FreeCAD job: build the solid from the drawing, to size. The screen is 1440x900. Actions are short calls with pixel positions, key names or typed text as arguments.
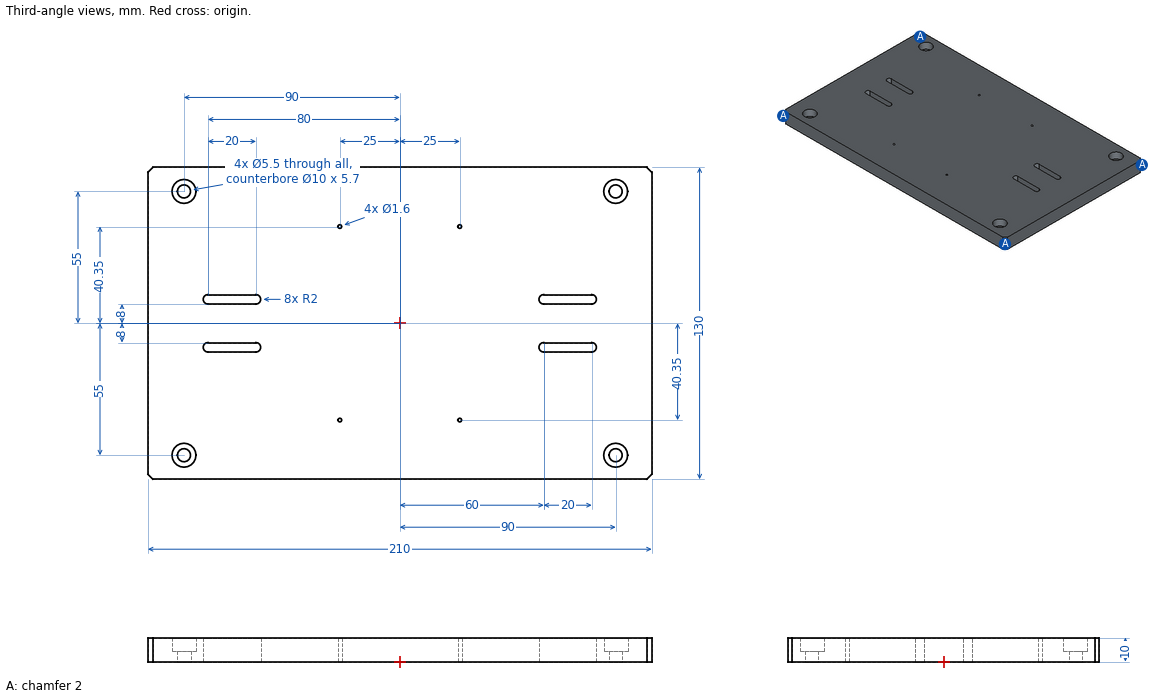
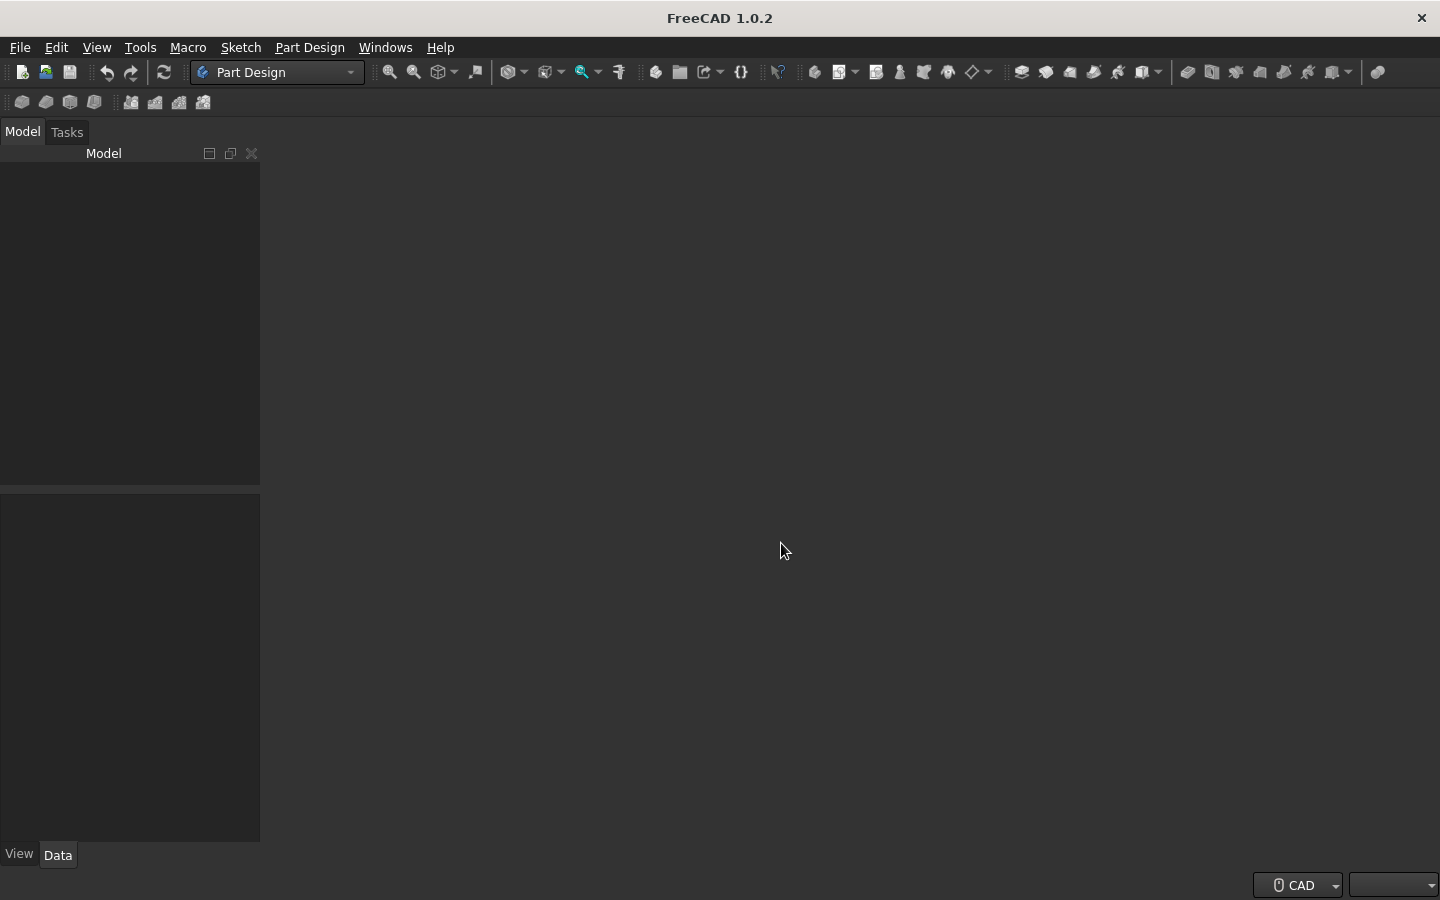
click(22, 72)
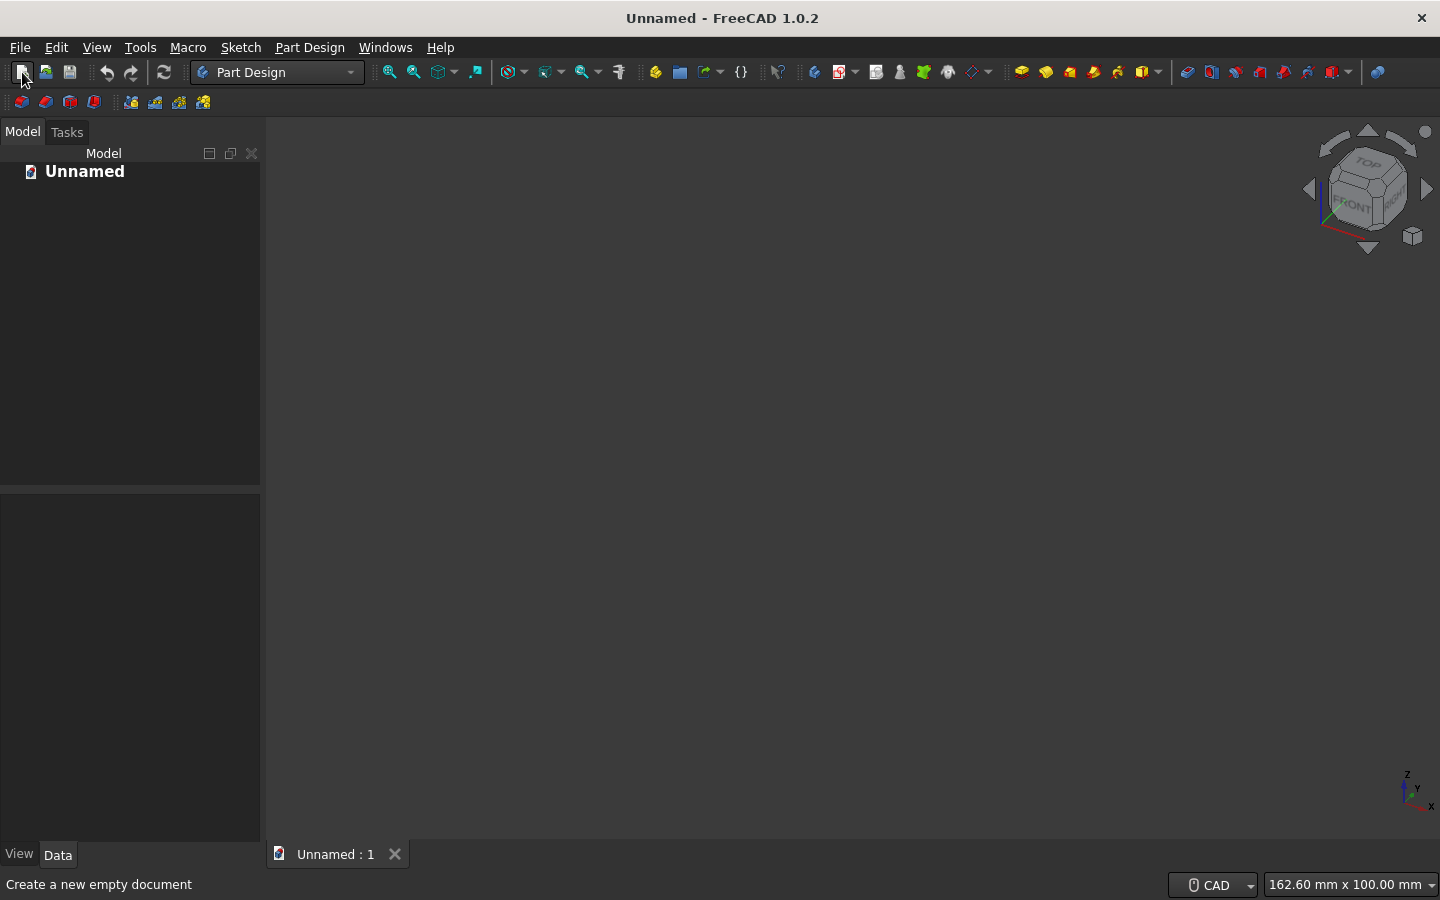
click(840, 72)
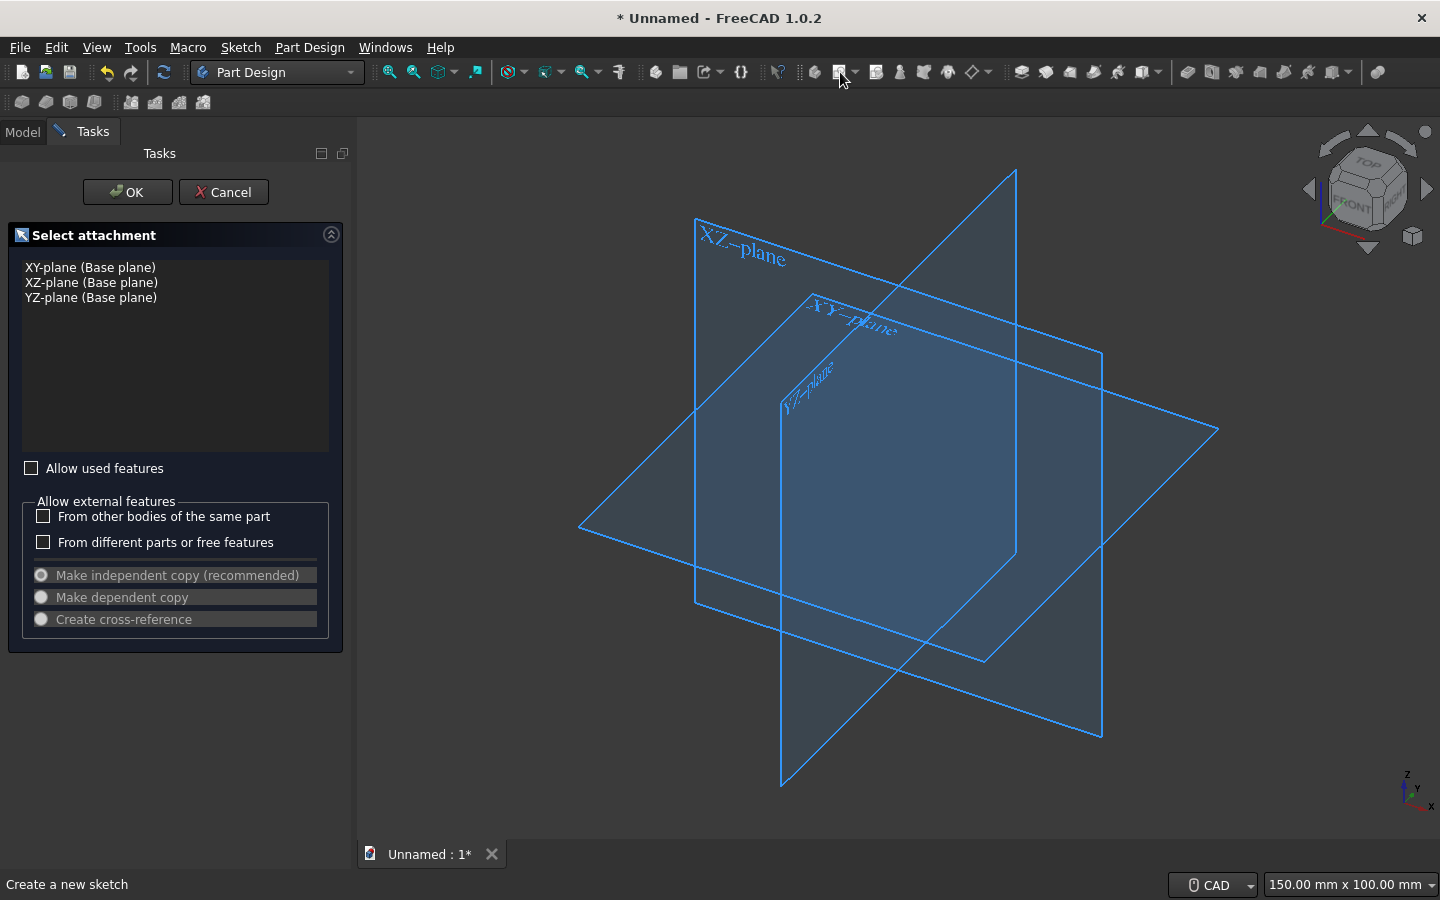
click(82, 268)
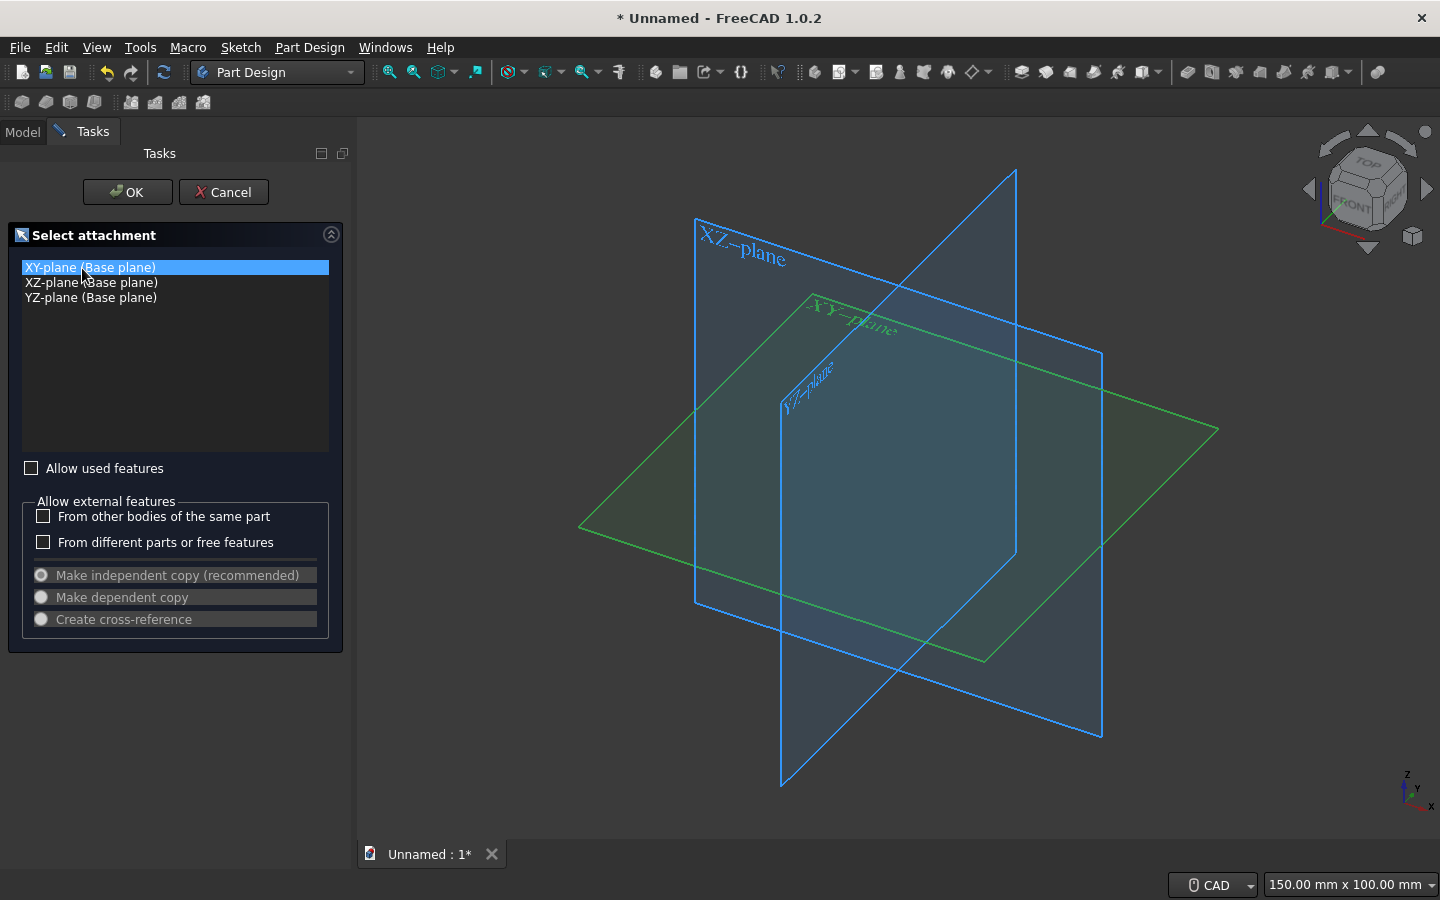
click(128, 192)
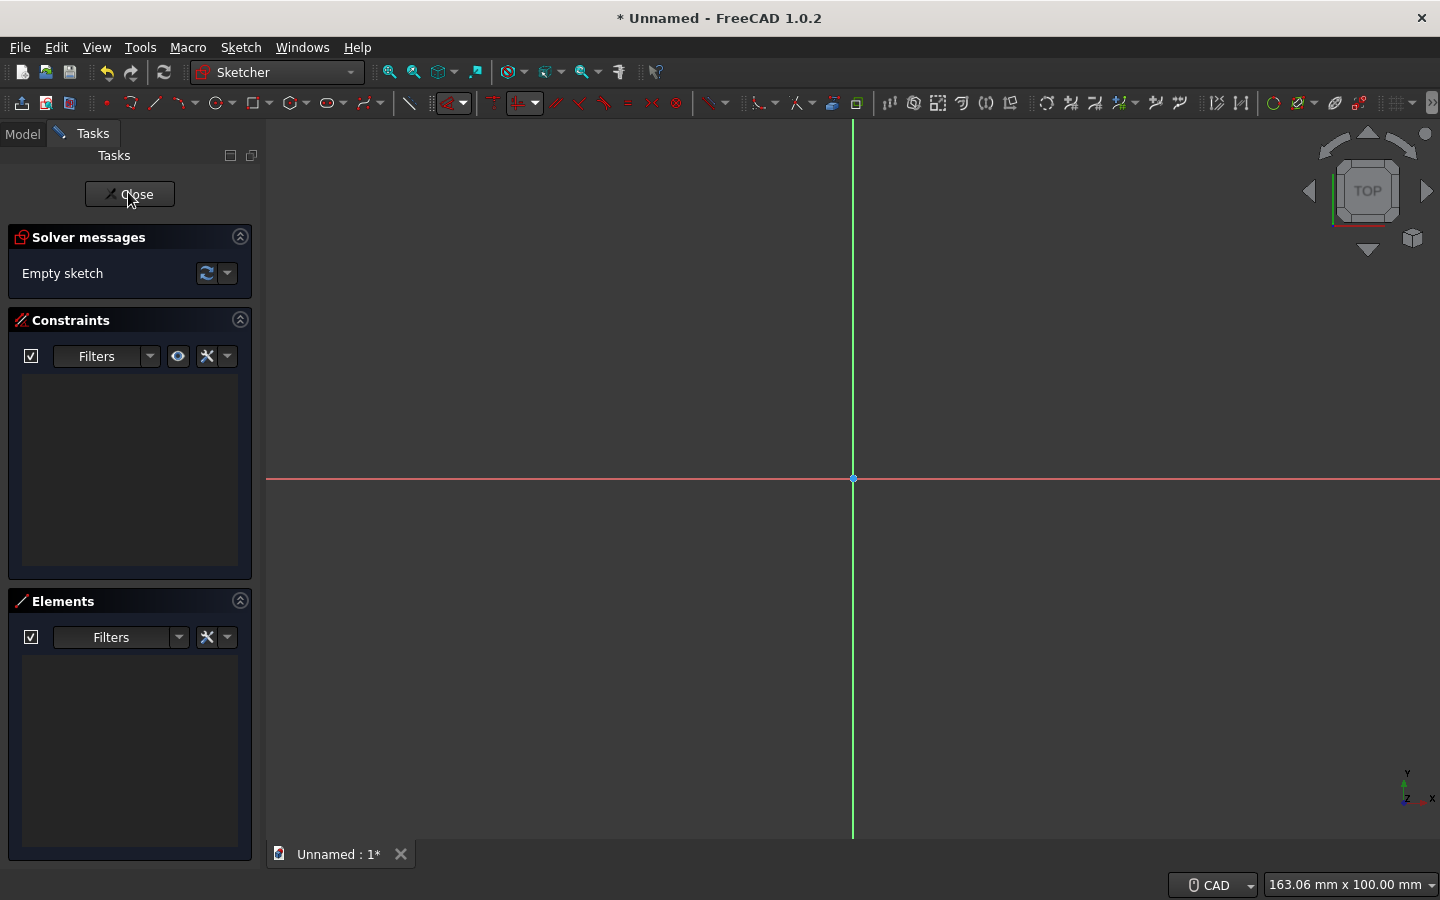
scroll(729, 479, down, 4)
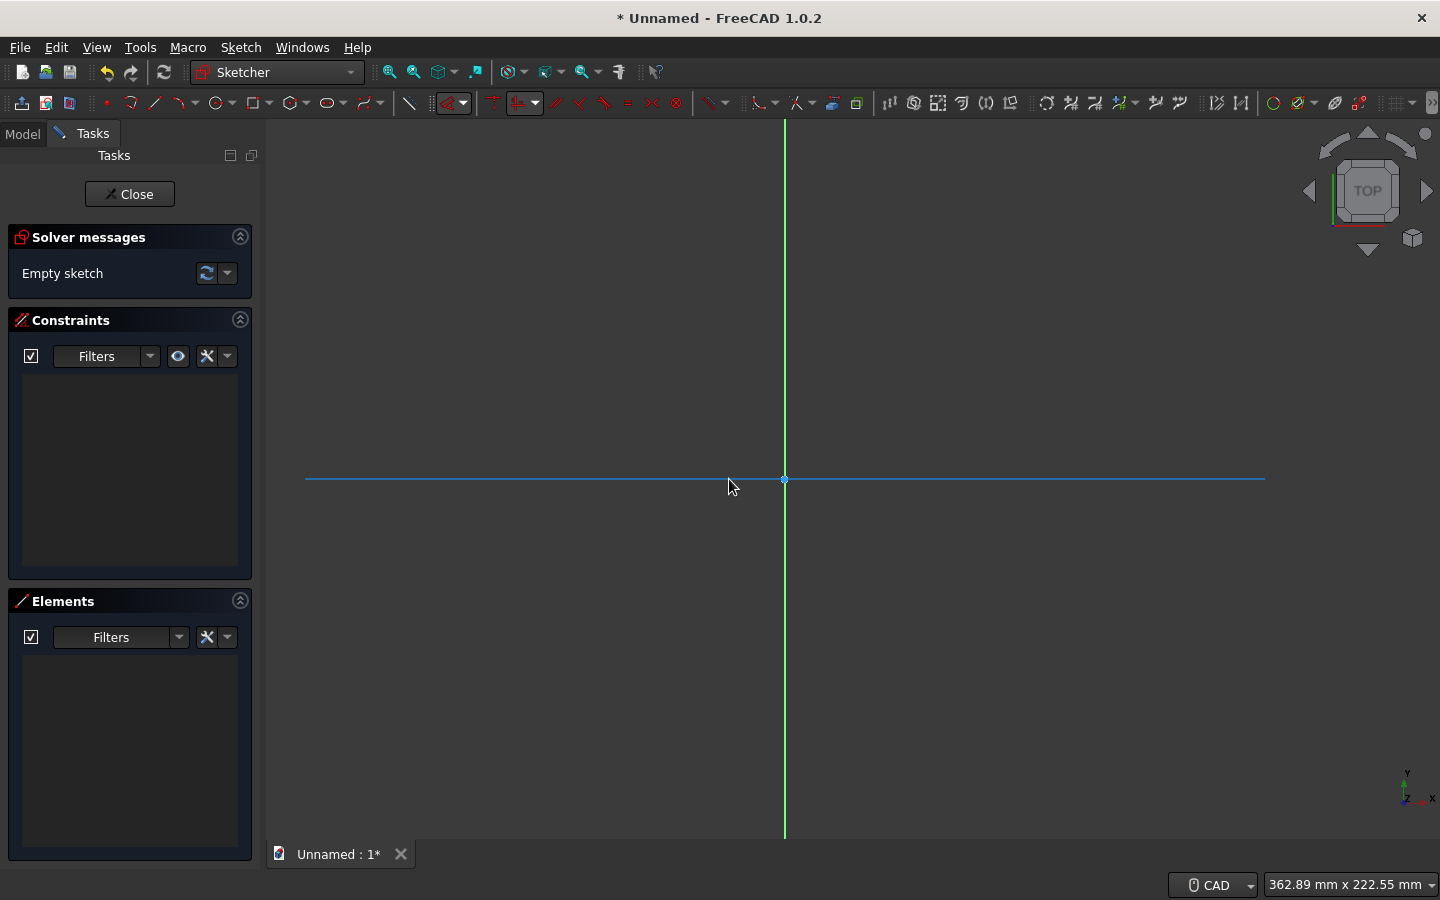
click(272, 104)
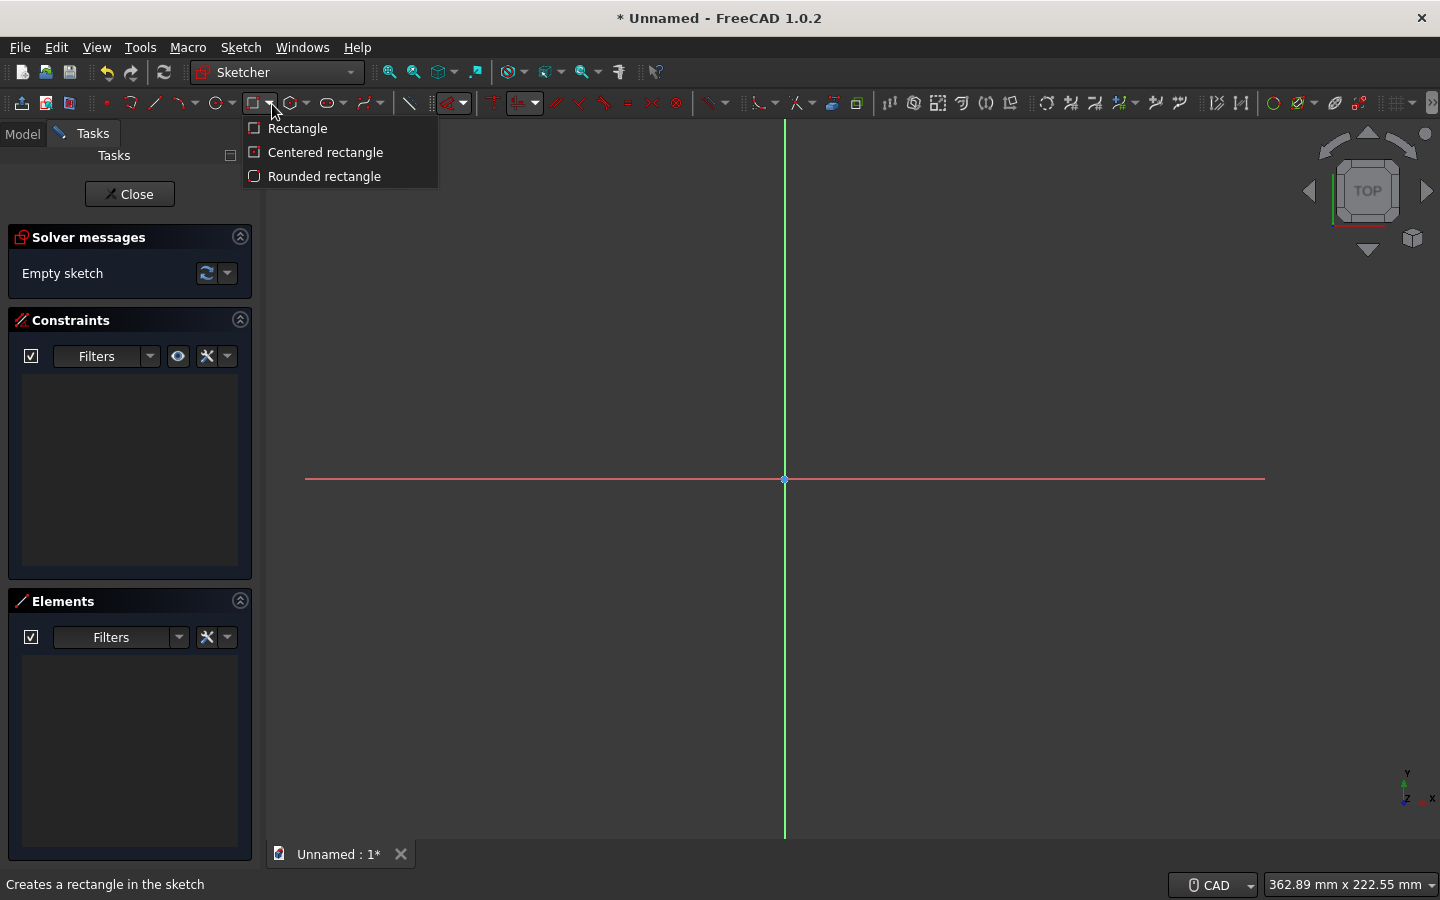
click(340, 152)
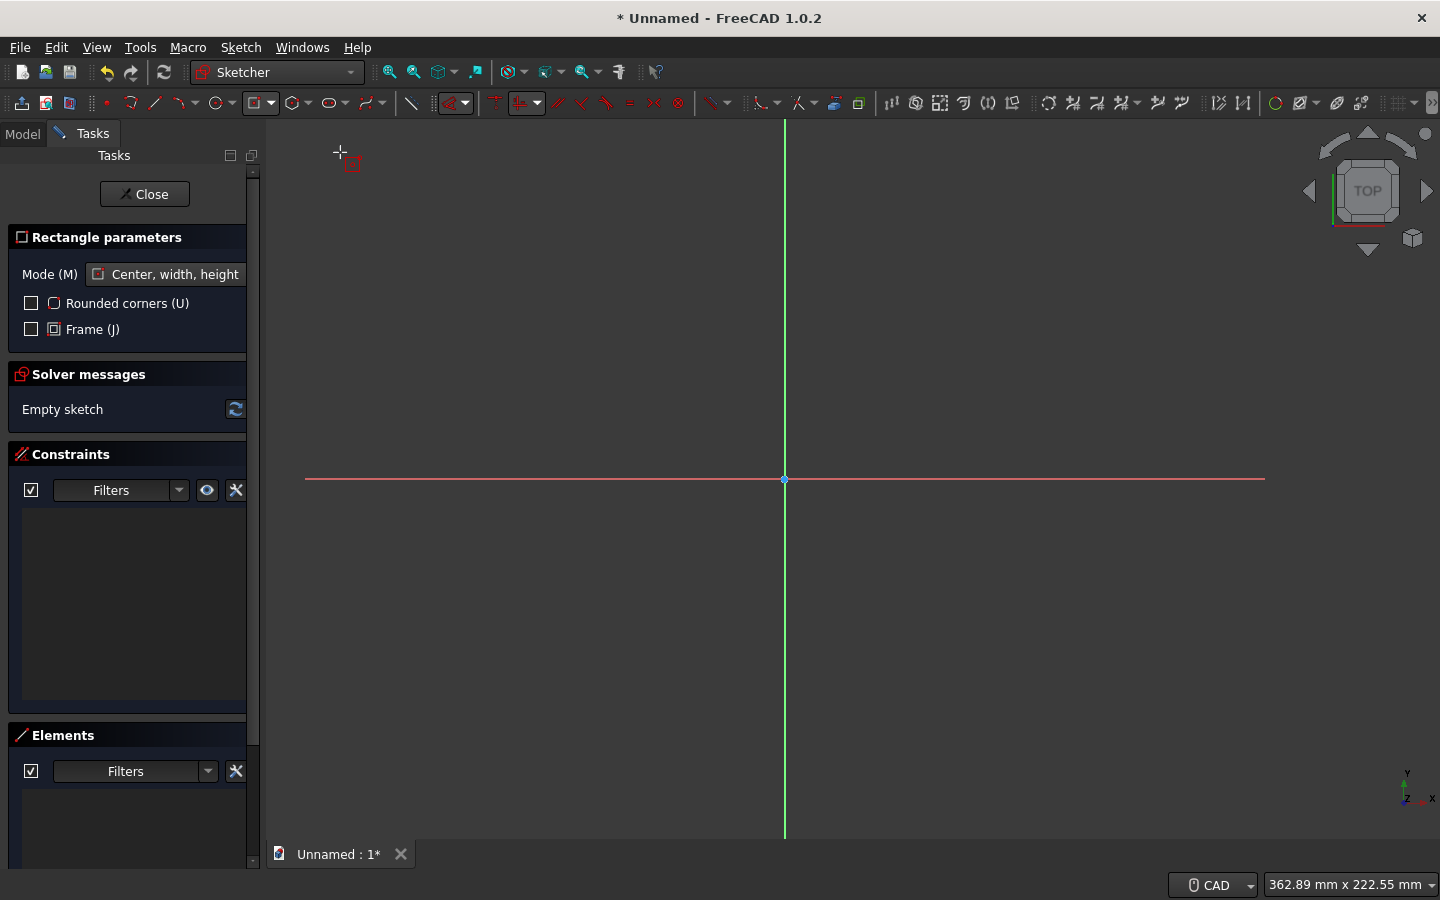
click(785, 479)
move(1125, 269)